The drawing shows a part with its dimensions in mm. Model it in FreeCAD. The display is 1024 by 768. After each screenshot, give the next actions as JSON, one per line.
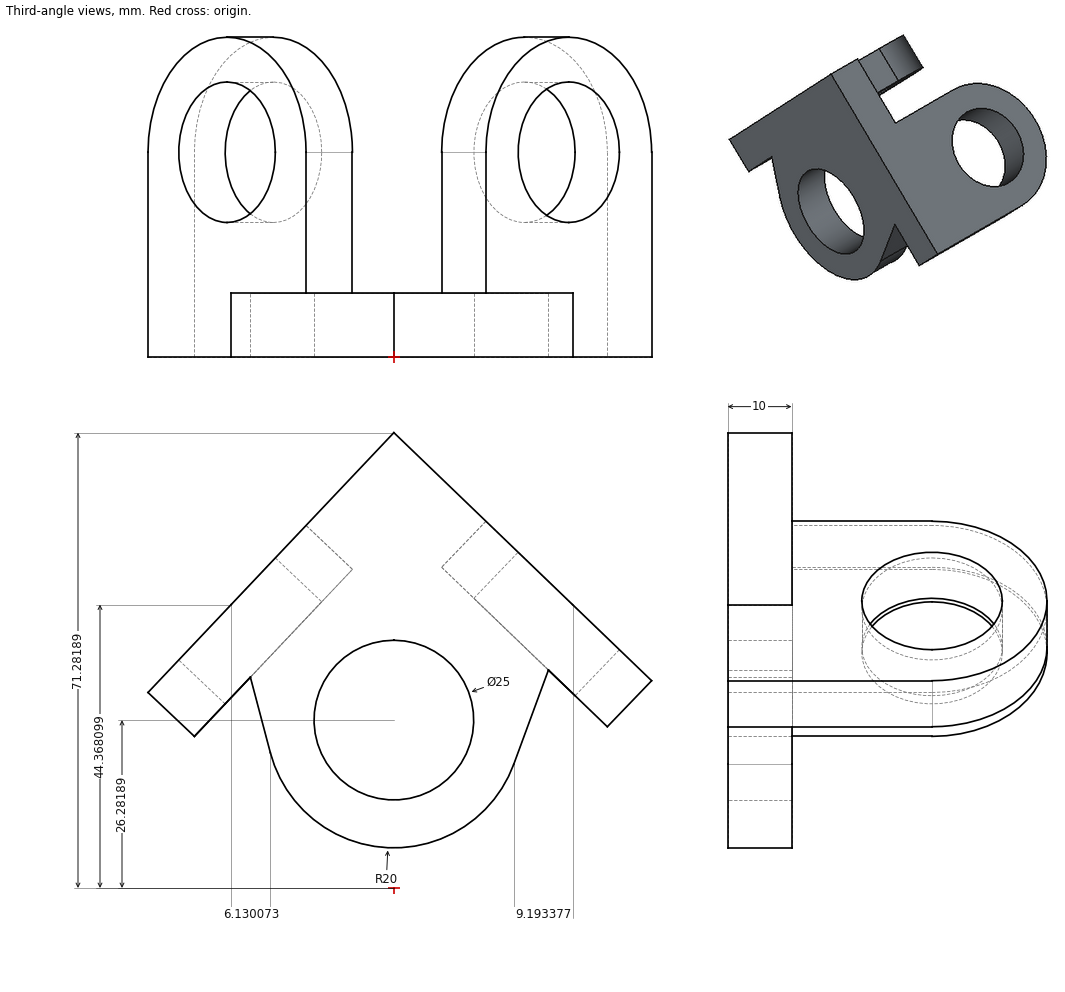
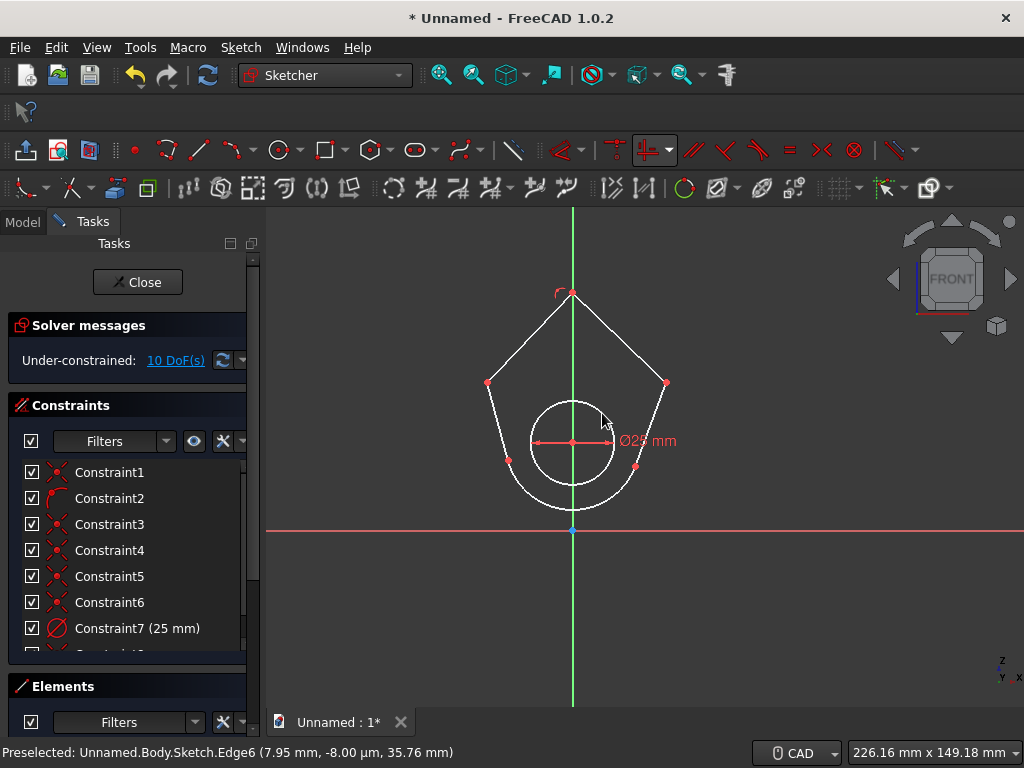
{"action": "left_click", "coordinate": [502, 438]}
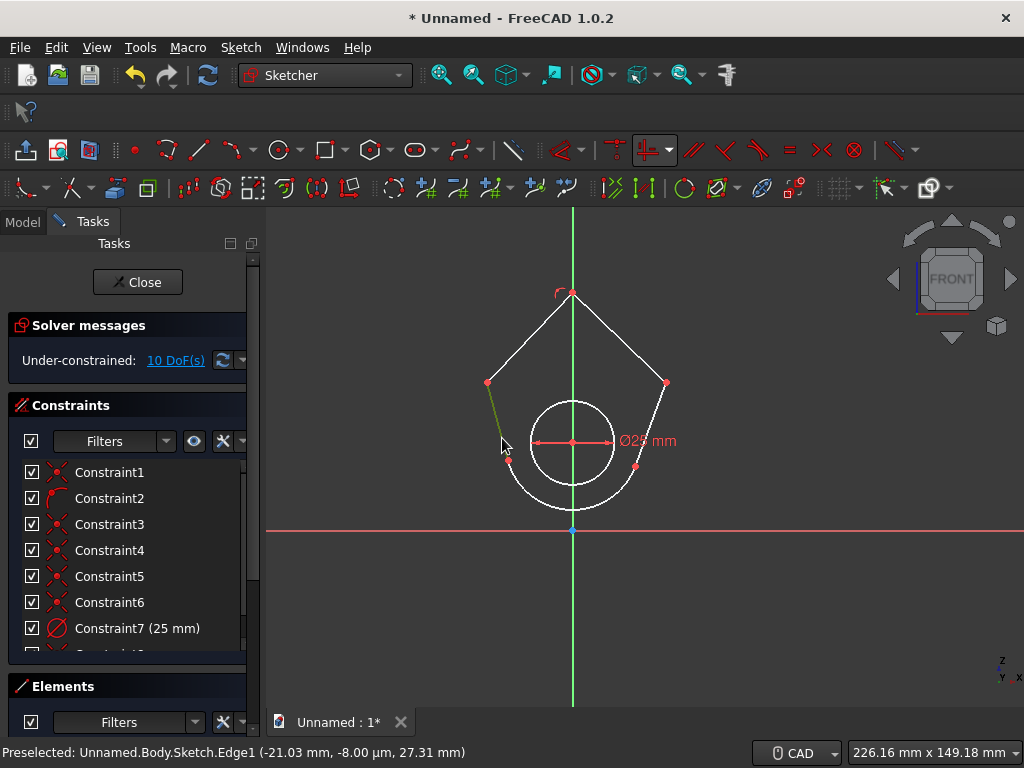
{"action": "left_click", "coordinate": [538, 500]}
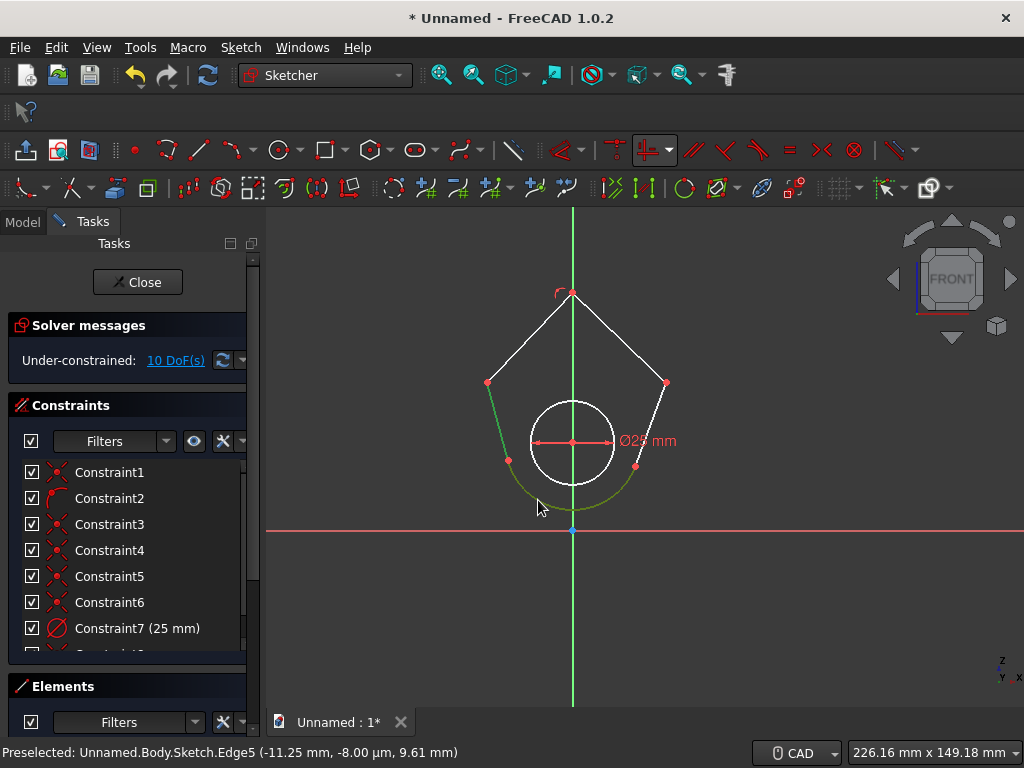
{"action": "left_click", "coordinate": [758, 150]}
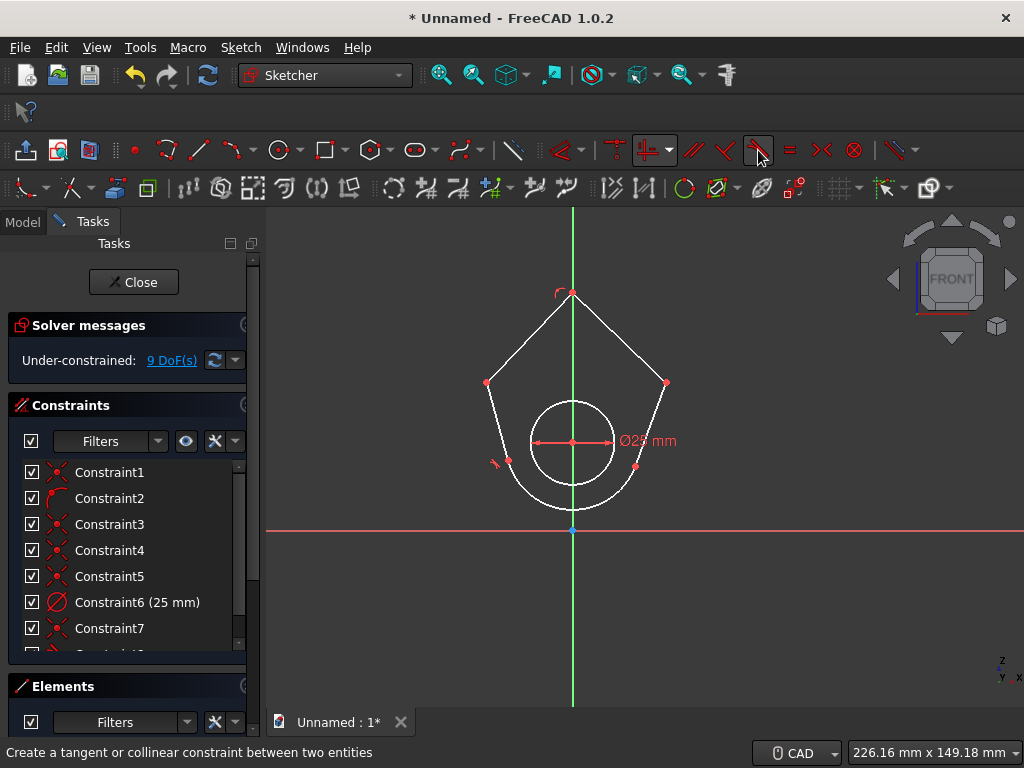
{"action": "left_click", "coordinate": [657, 408]}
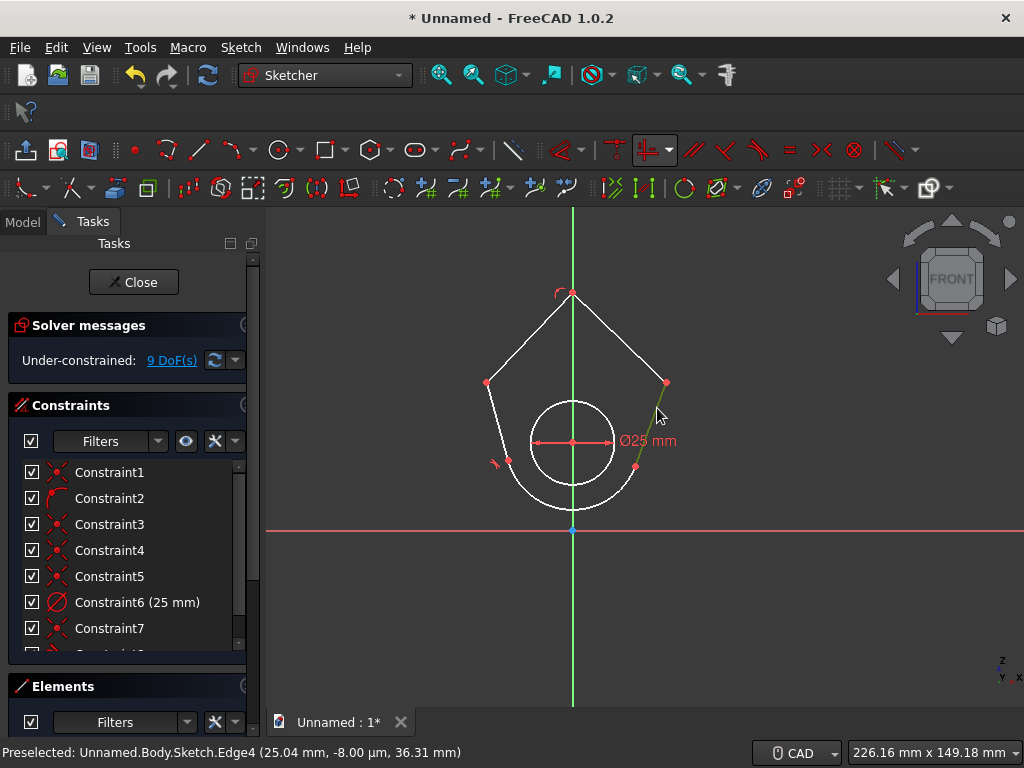
{"action": "left_click", "coordinate": [537, 500]}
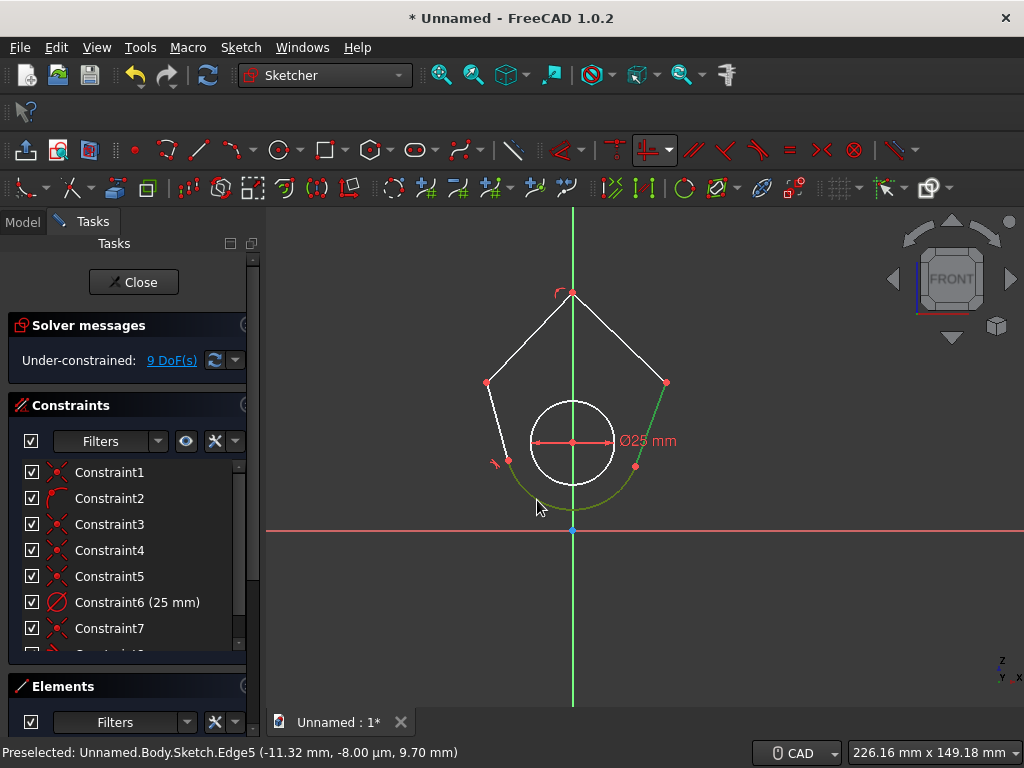
{"action": "left_click", "coordinate": [758, 150]}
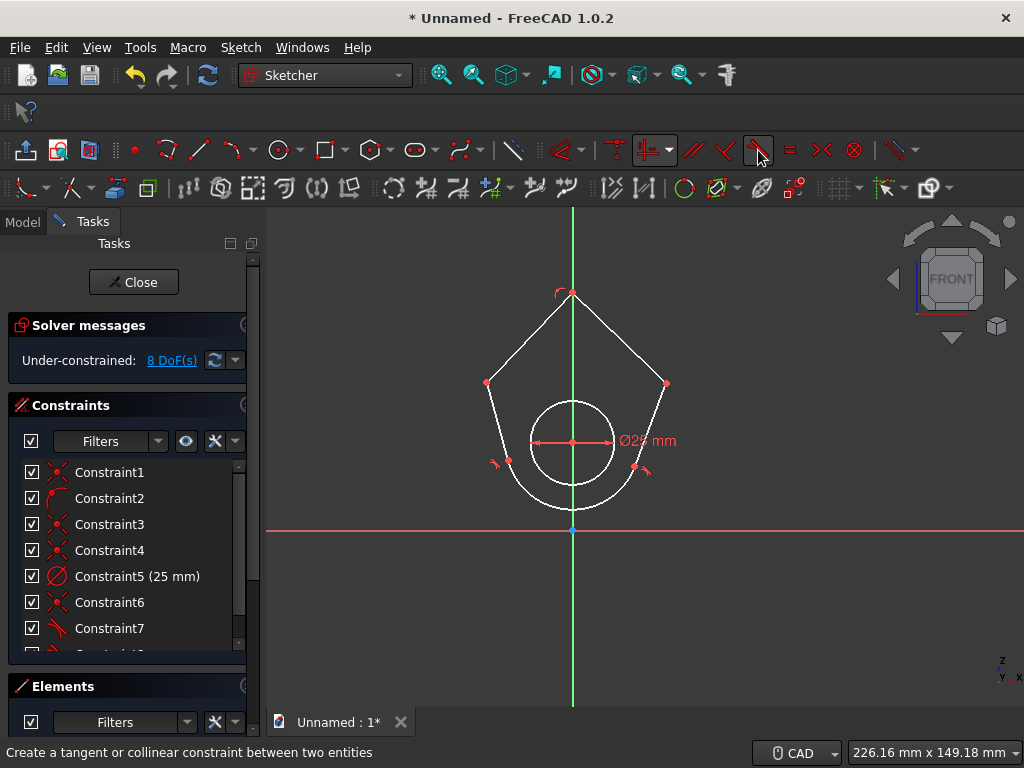
{"action": "left_click", "coordinate": [572, 443]}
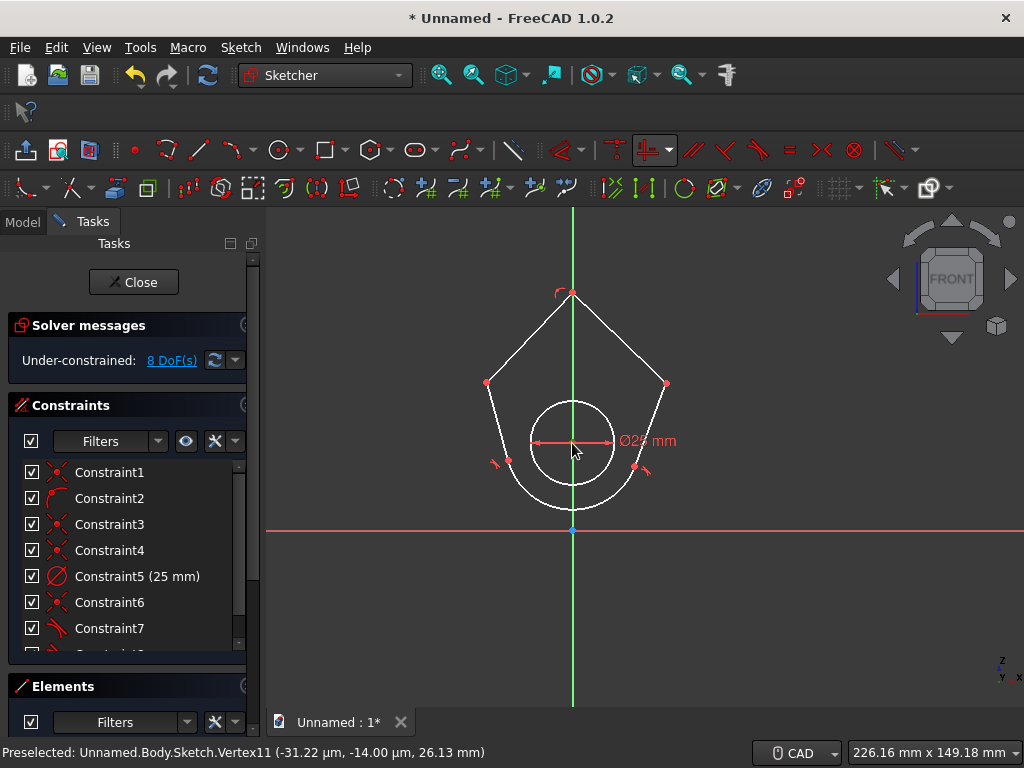
{"action": "left_click", "coordinate": [573, 647]}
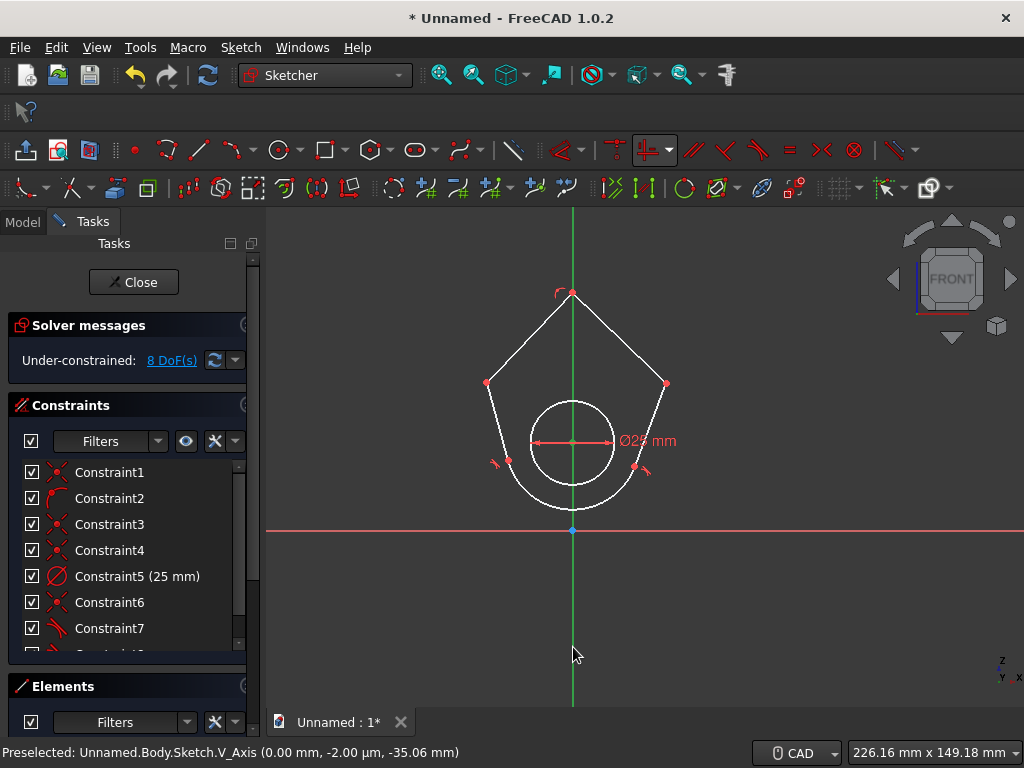
{"action": "left_click", "coordinate": [616, 150]}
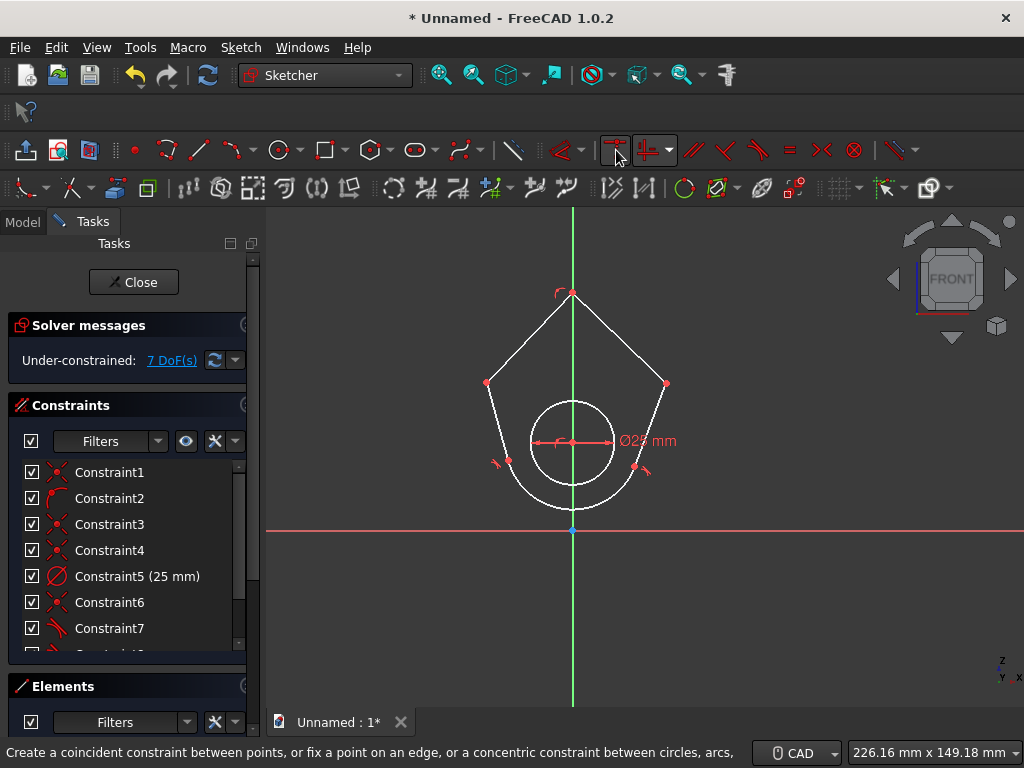
{"action": "left_click", "coordinate": [538, 500]}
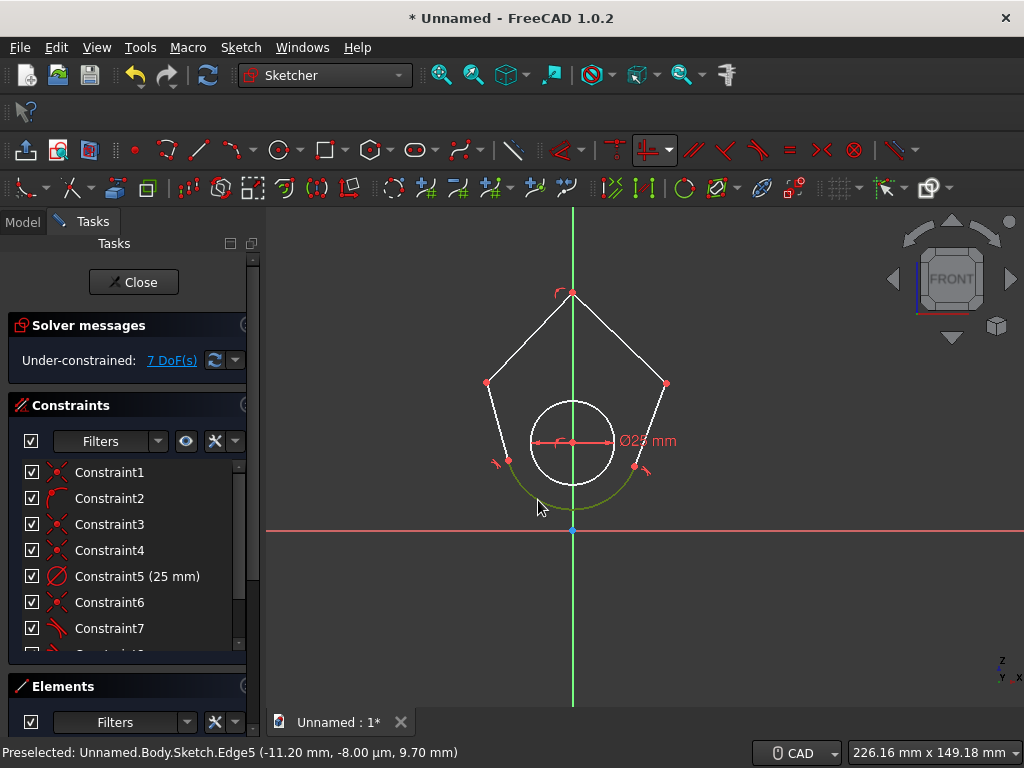
{"action": "key", "text": "k r"}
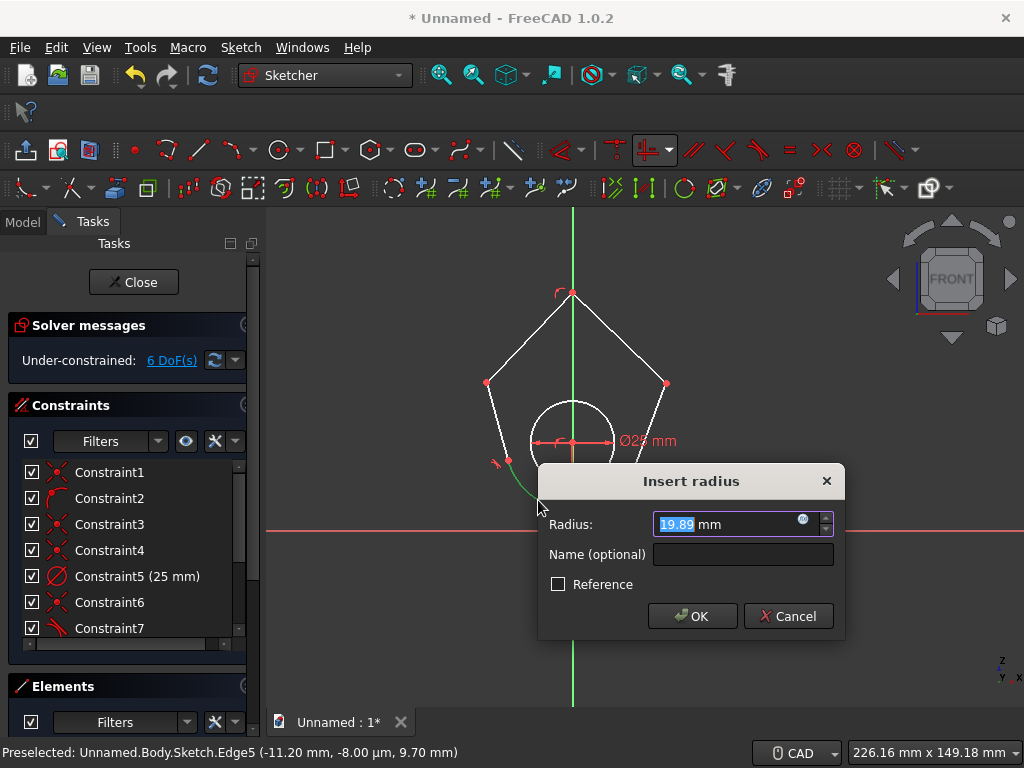
{"action": "type", "text": "20"}
{"action": "key", "text": "Return"}